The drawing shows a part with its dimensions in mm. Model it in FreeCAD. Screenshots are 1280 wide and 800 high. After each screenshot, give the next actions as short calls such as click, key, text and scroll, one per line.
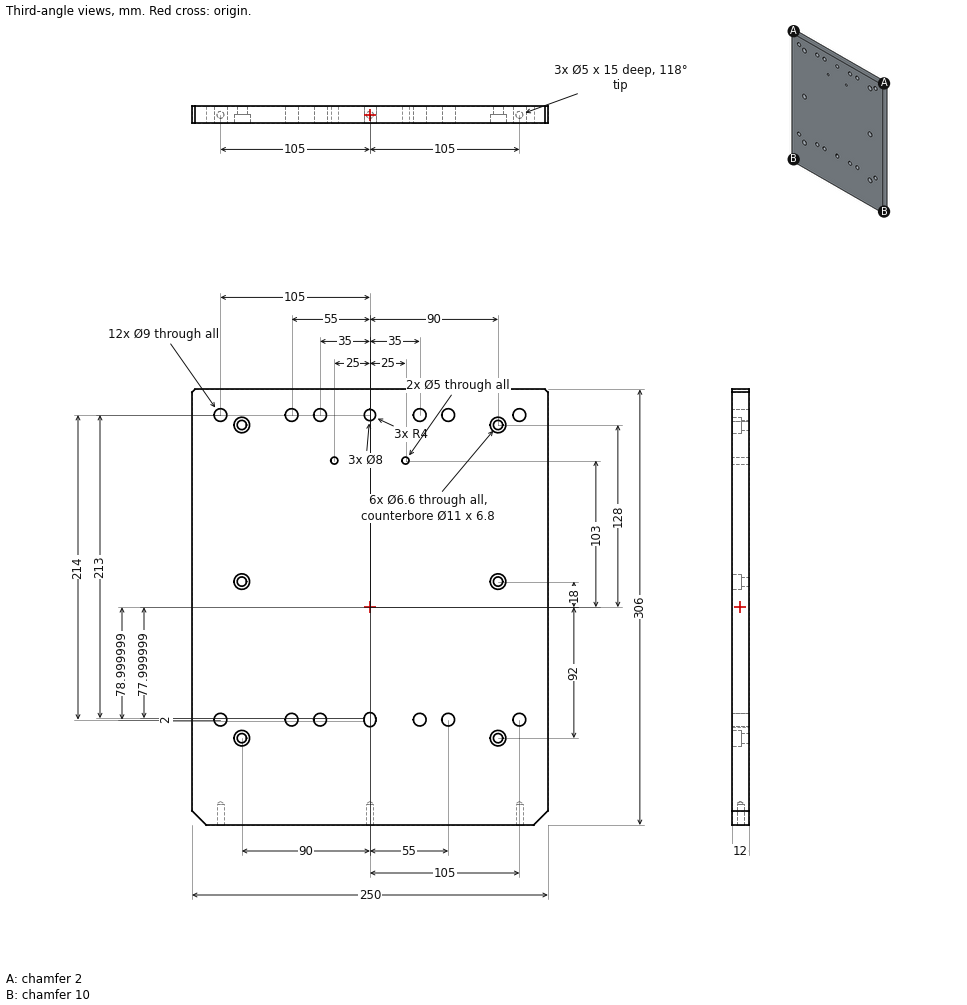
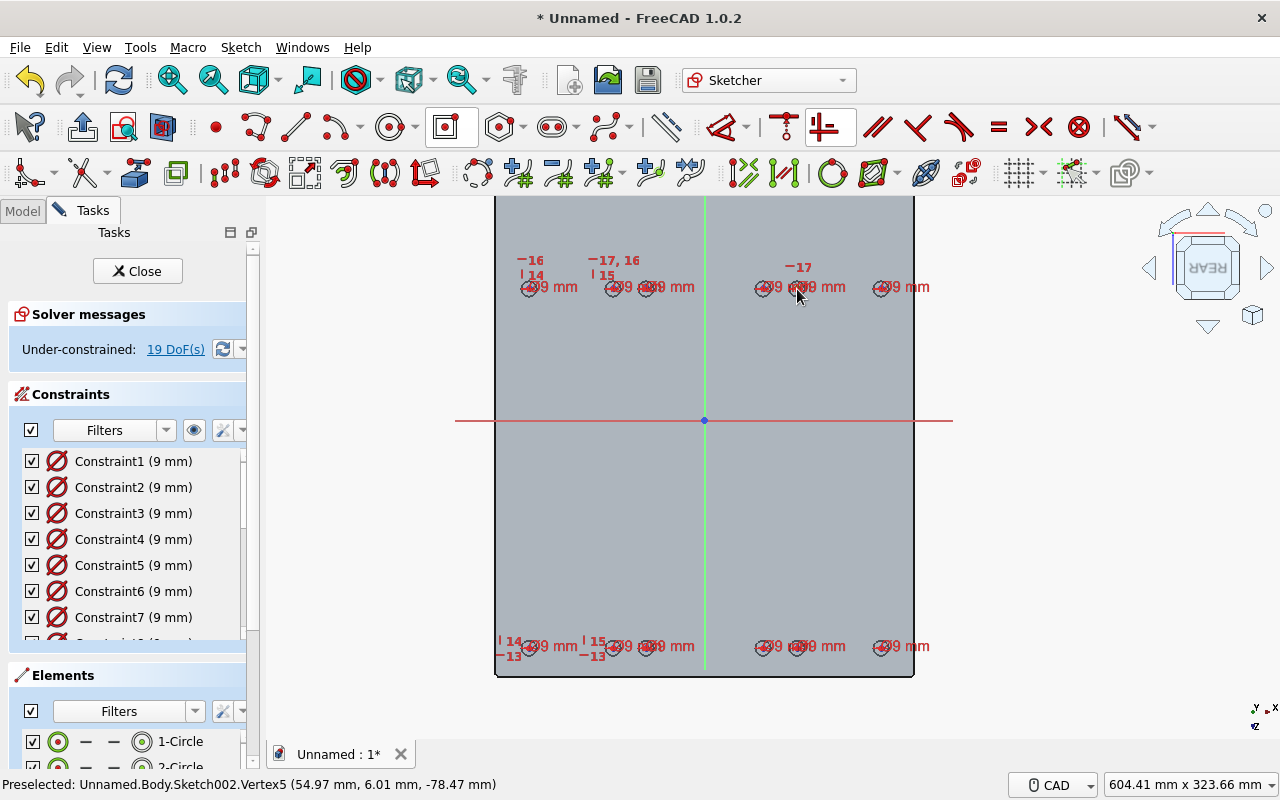
click(881, 289)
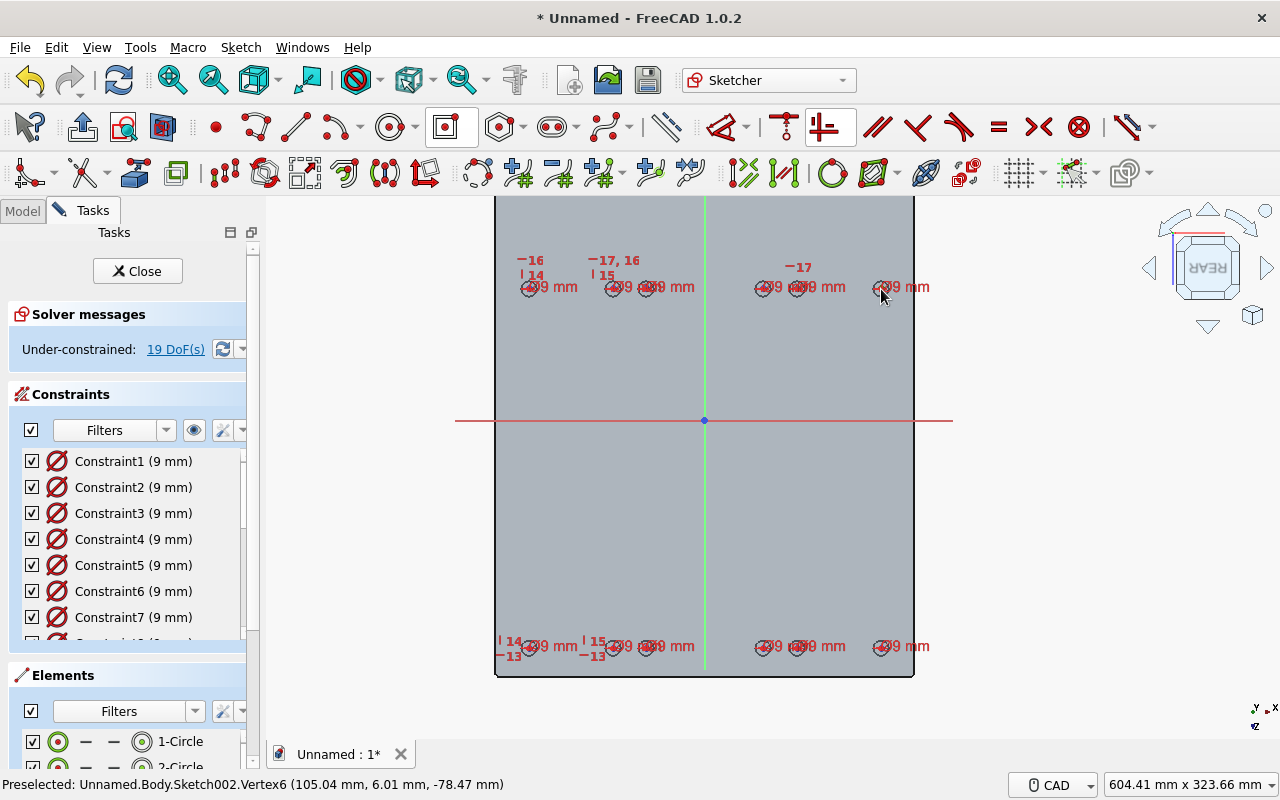
key(h)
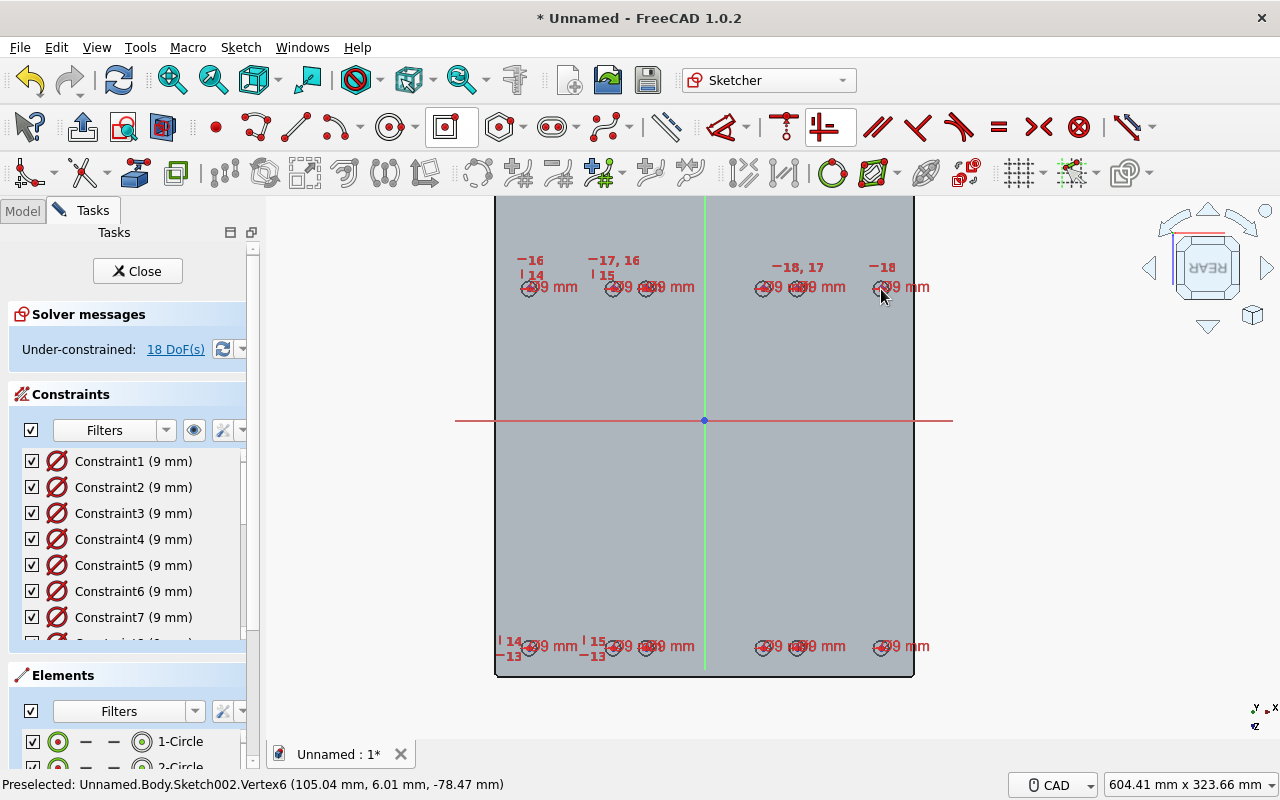
click(797, 289)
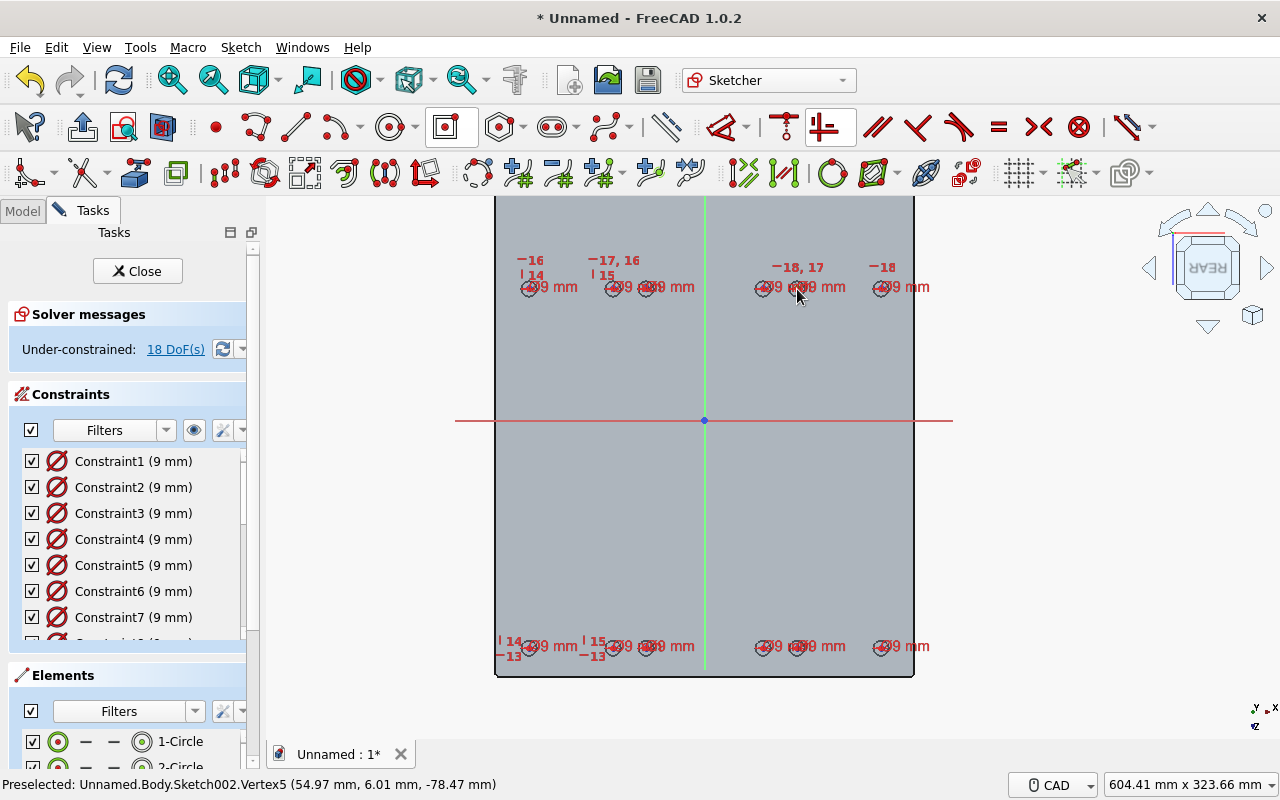
click(797, 648)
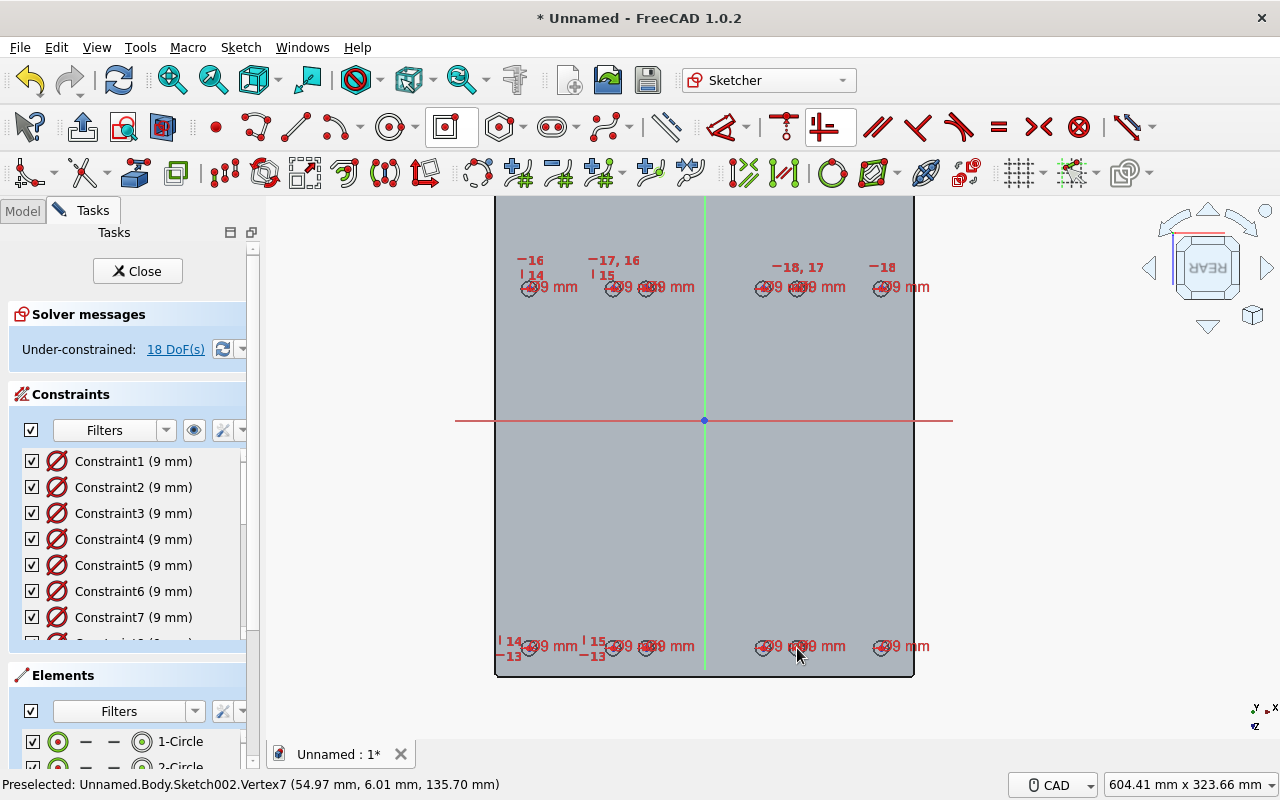
key(v)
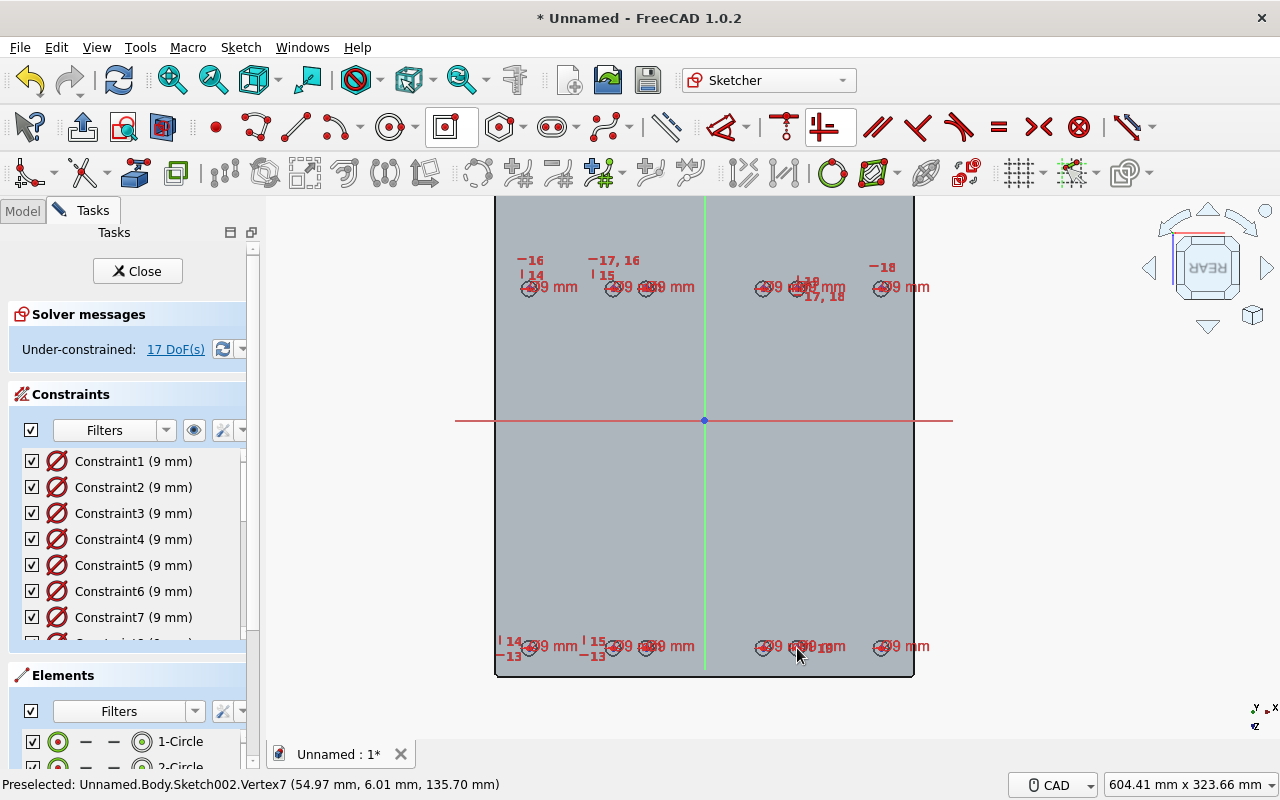
click(613, 648)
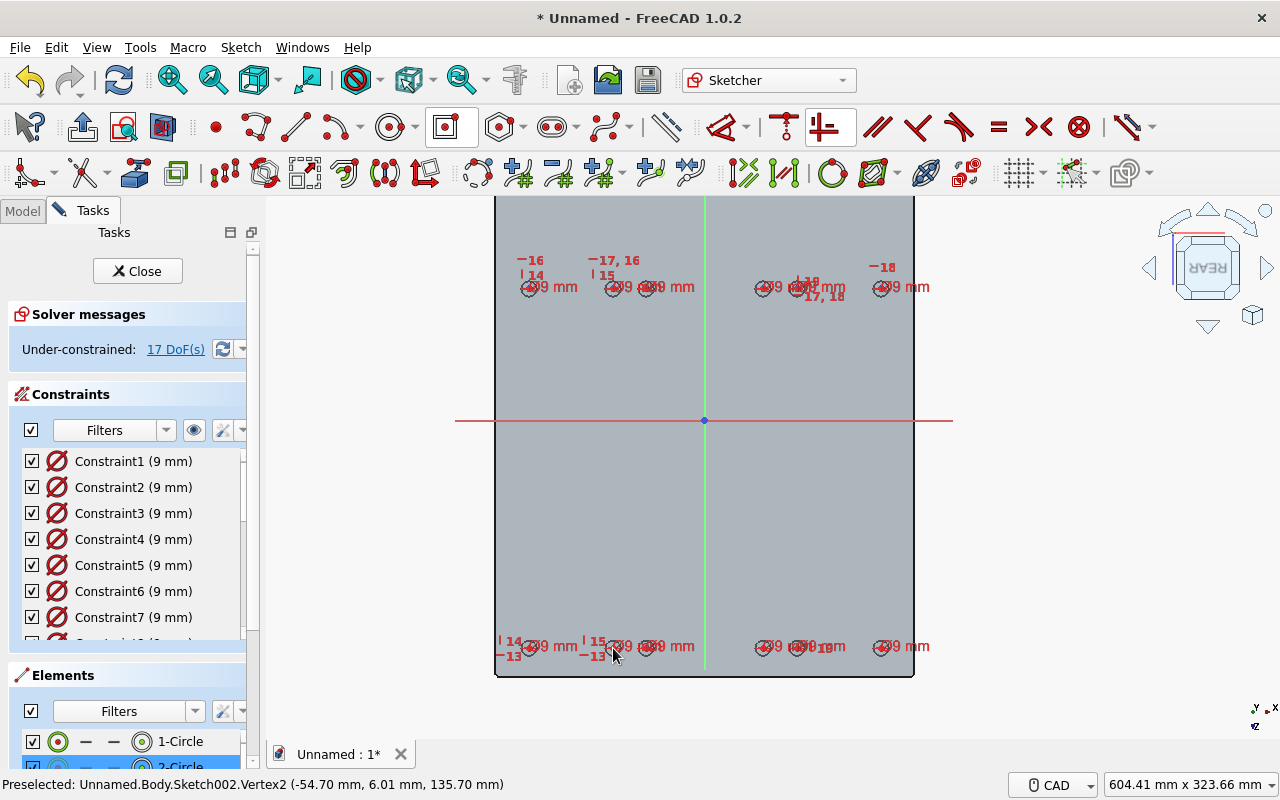
click(797, 648)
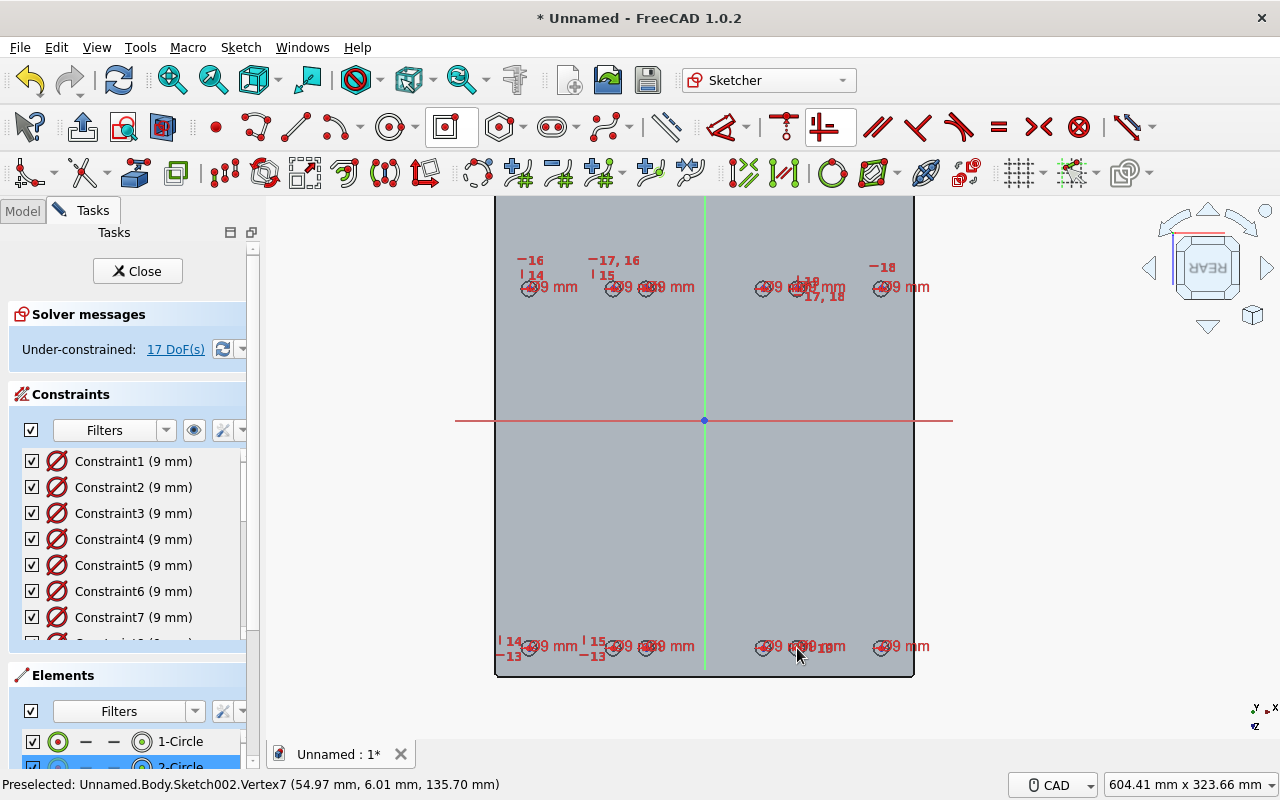
click(850, 128)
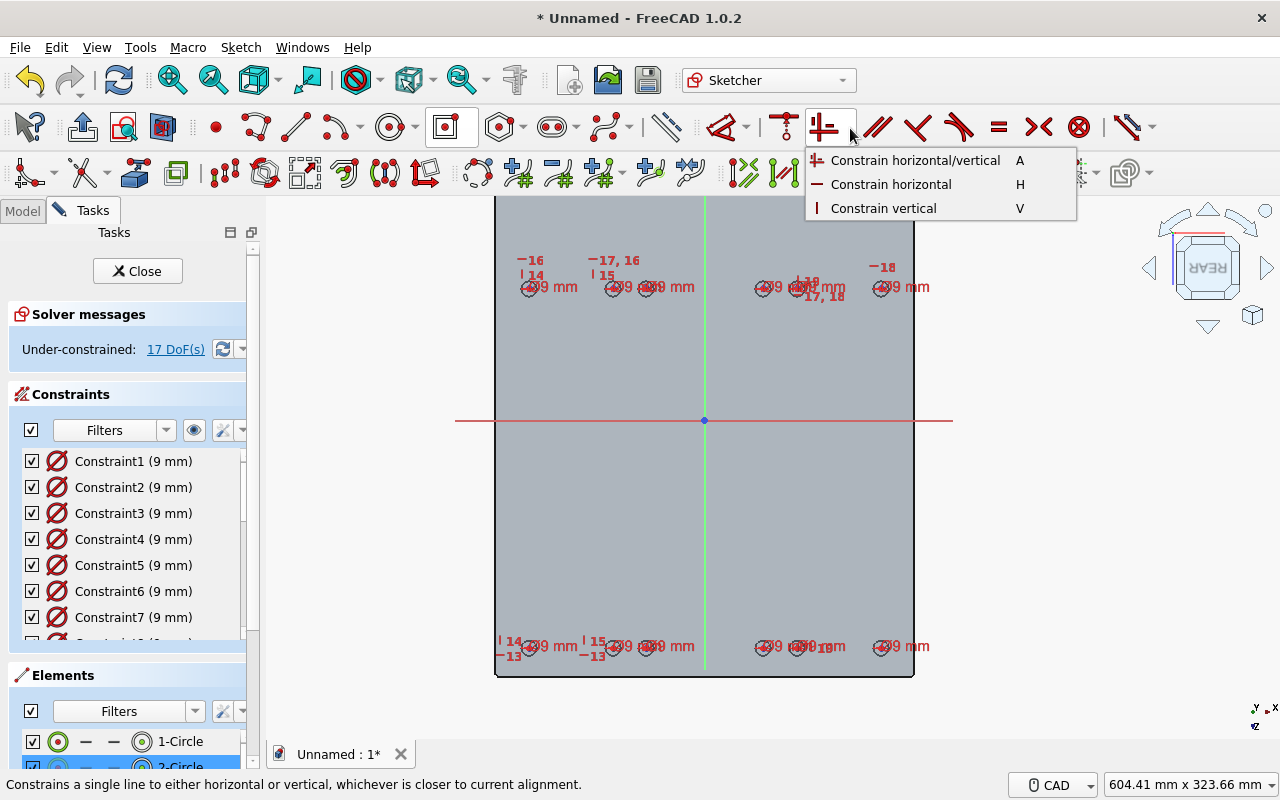
click(941, 184)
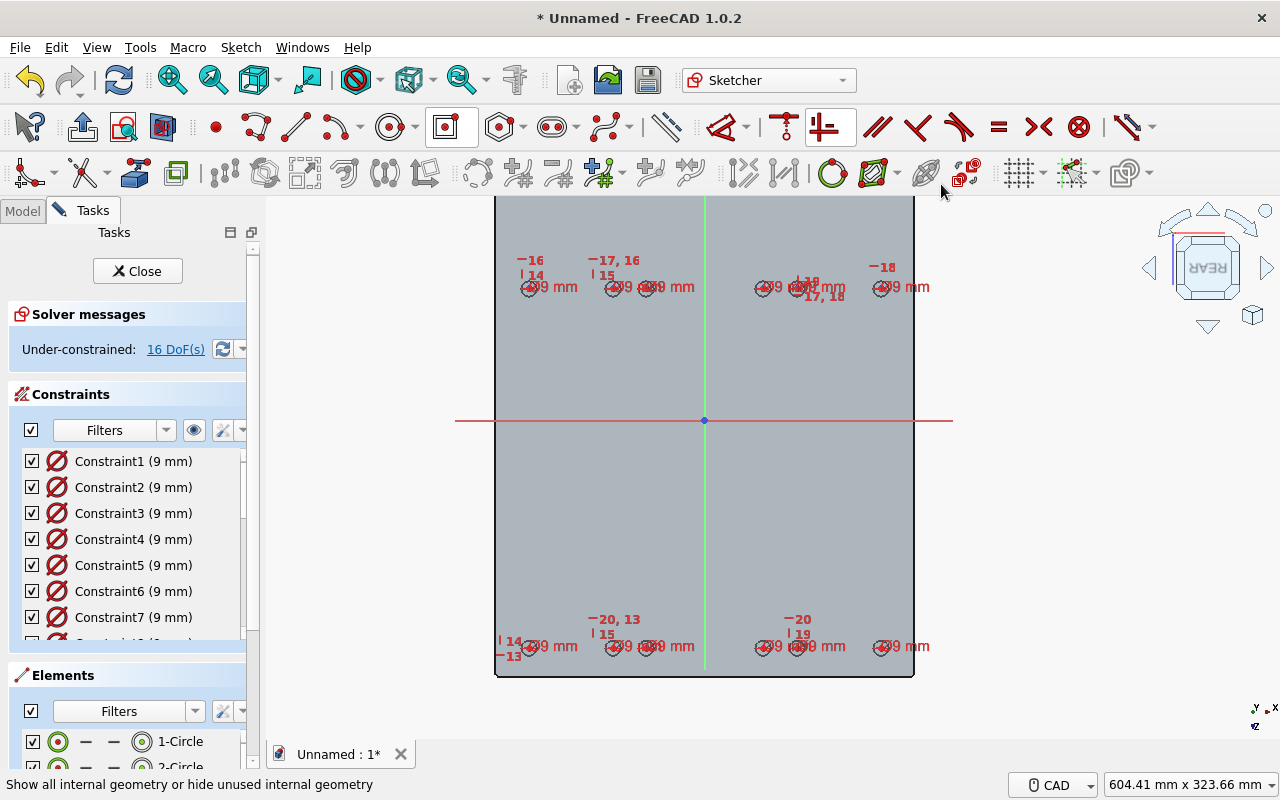
click(881, 289)